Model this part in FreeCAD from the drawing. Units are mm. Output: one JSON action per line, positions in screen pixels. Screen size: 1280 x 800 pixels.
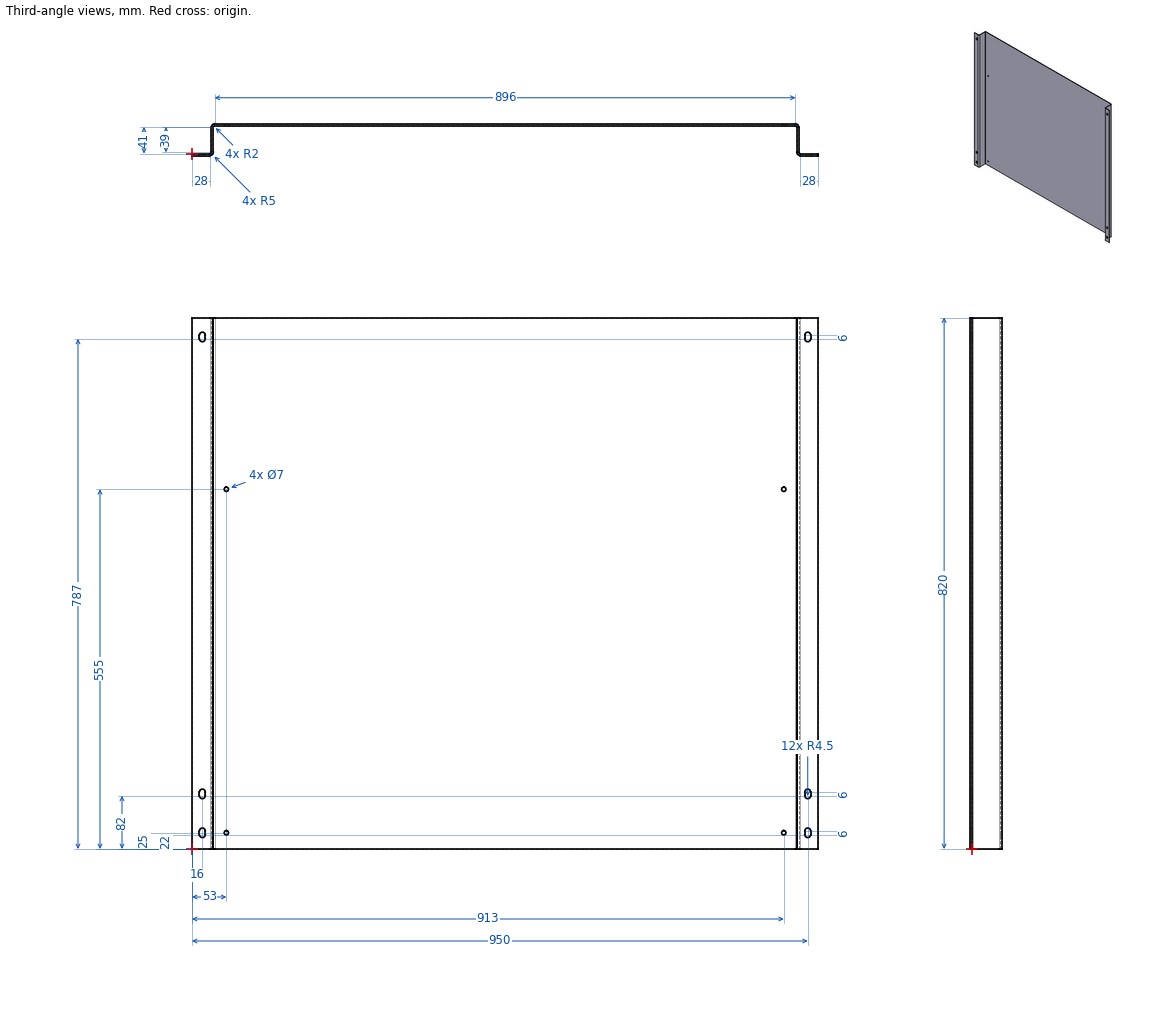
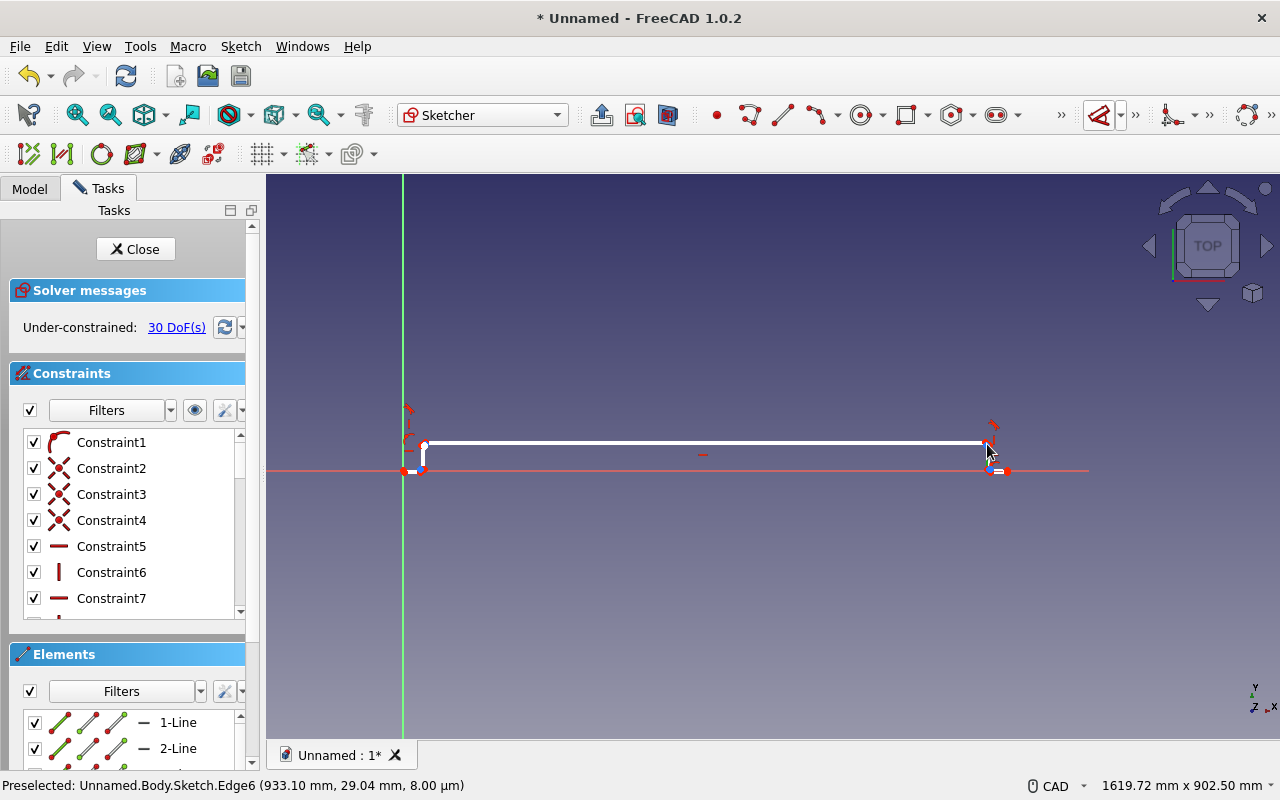
{"action": "scroll", "coordinate": [988, 471], "scroll_direction": "up", "scroll_amount": 12}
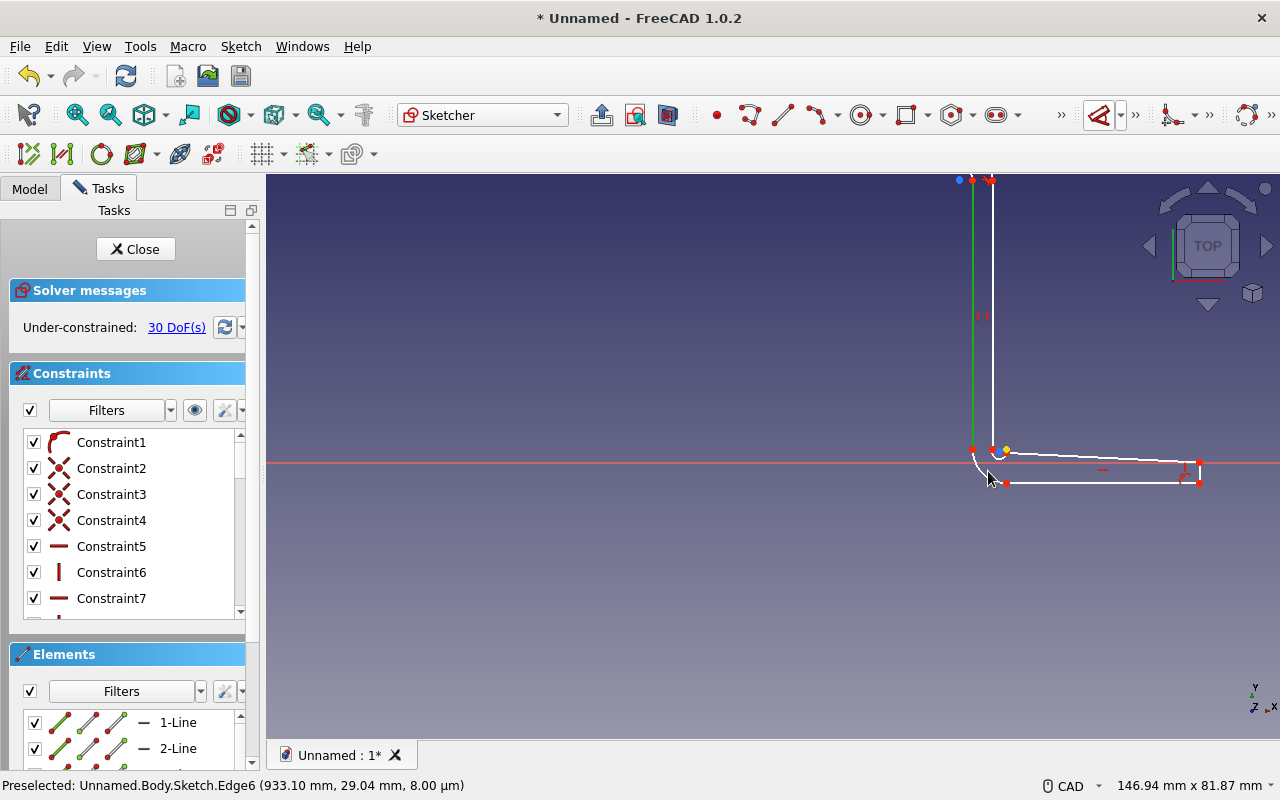
{"action": "left_click", "coordinate": [977, 465]}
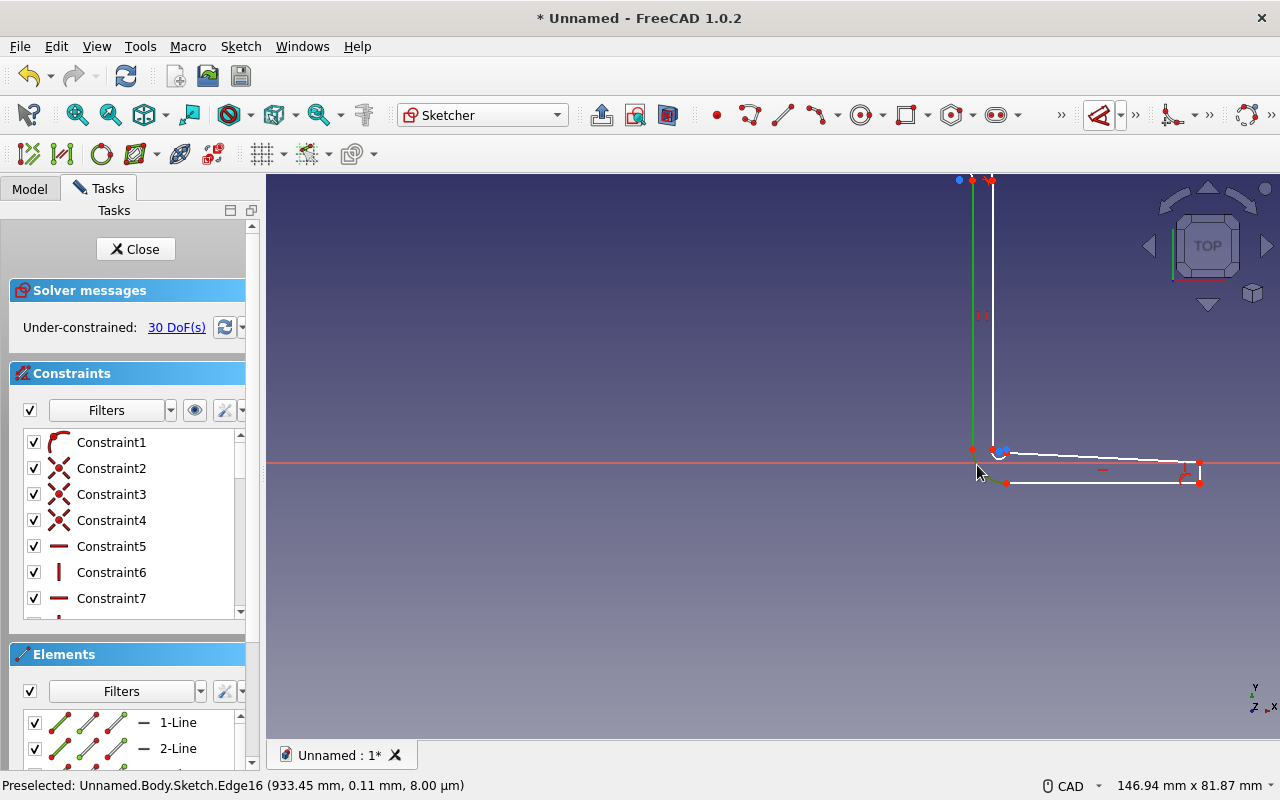
{"action": "key", "text": "t"}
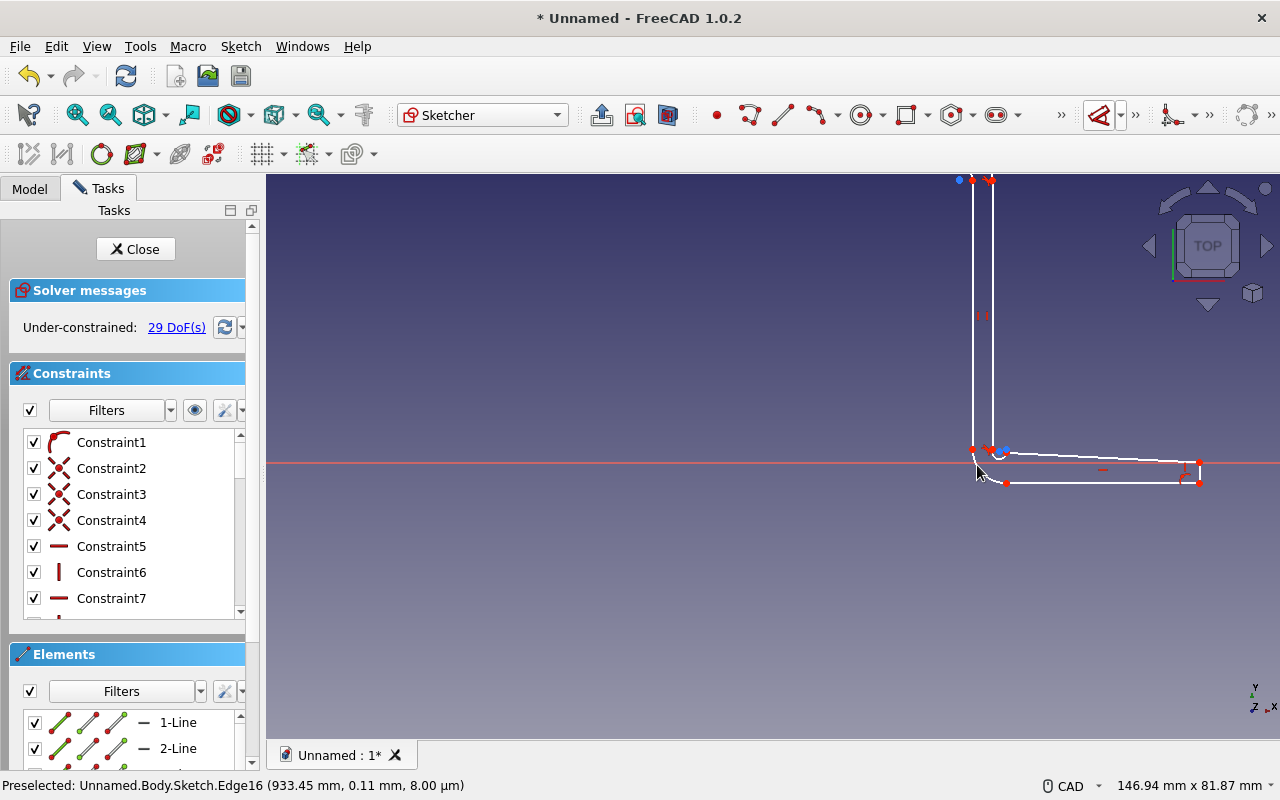
{"action": "left_click", "coordinate": [1064, 483]}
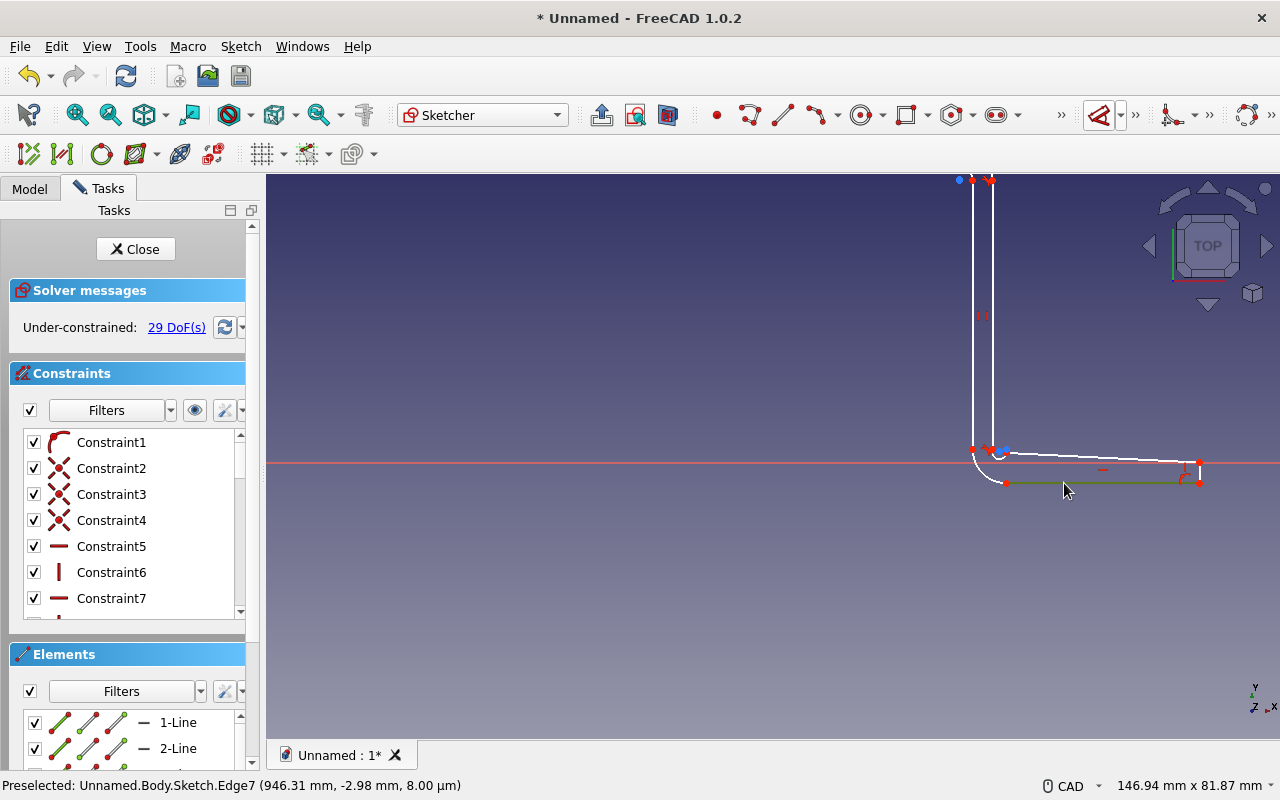
{"action": "left_click", "coordinate": [977, 465]}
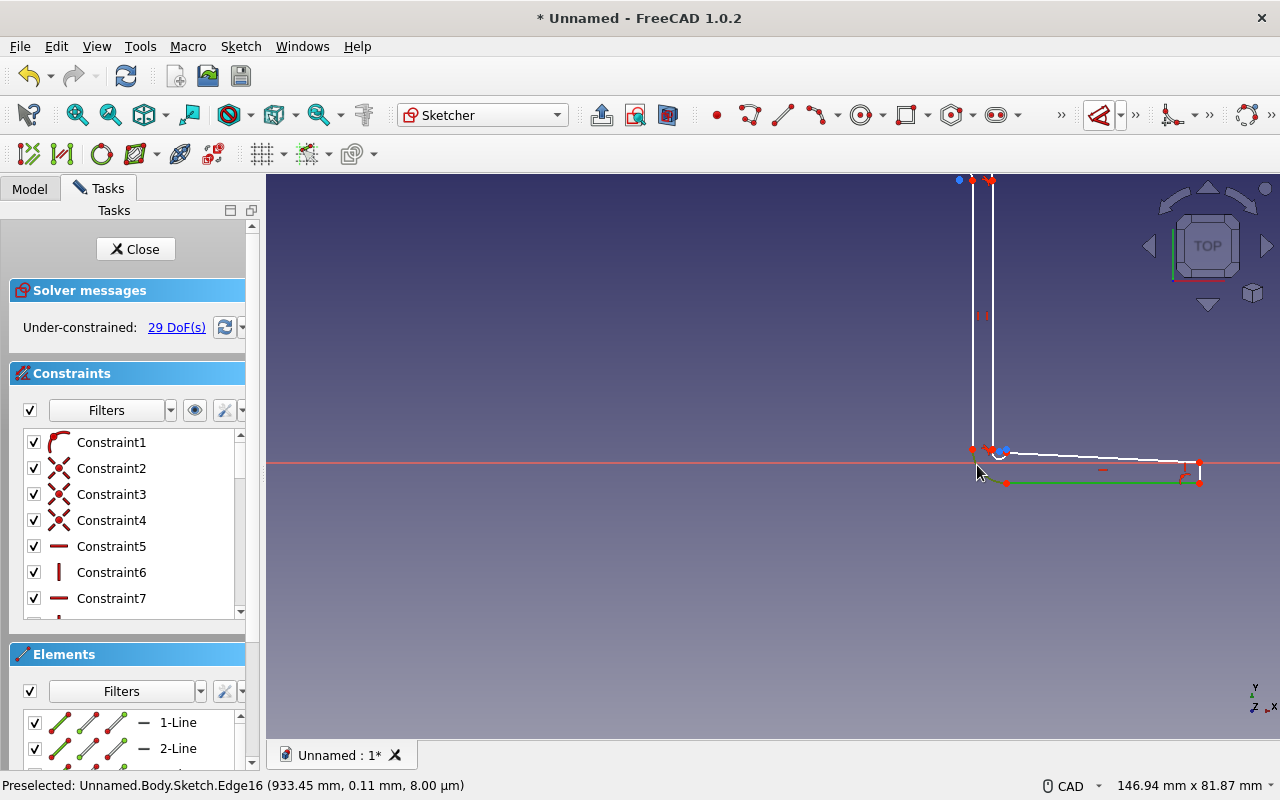
{"action": "key", "text": "t"}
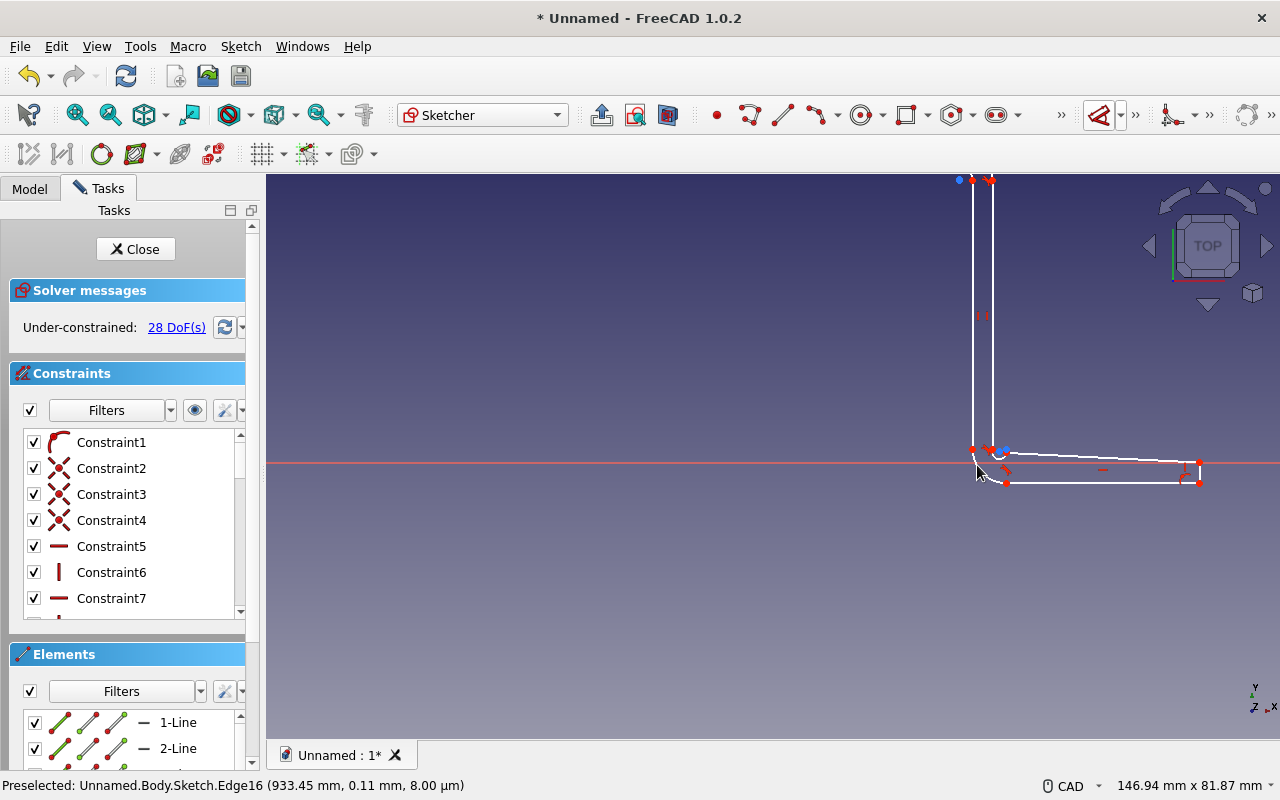
{"action": "scroll", "coordinate": [988, 471], "scroll_direction": "down", "scroll_amount": 12}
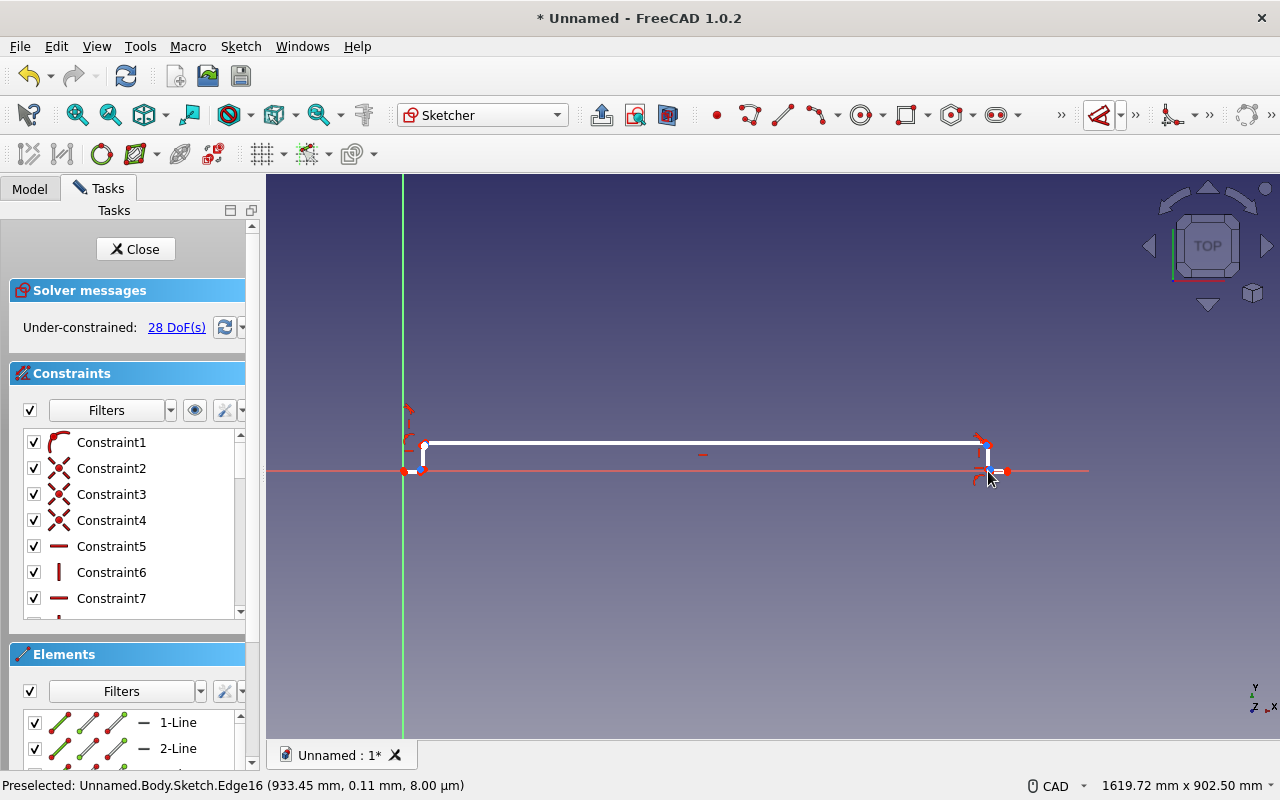
{"action": "scroll", "coordinate": [1003, 470], "scroll_direction": "up", "scroll_amount": 10}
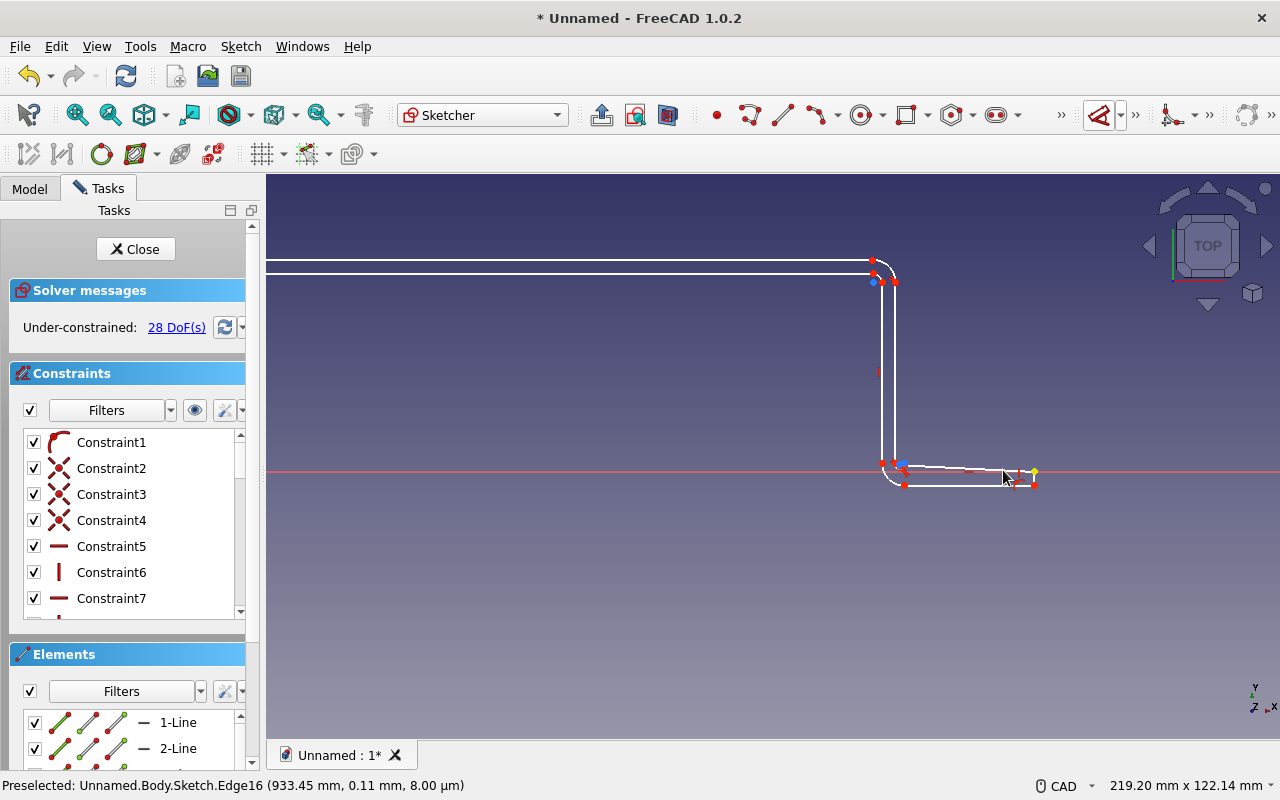
{"action": "left_click", "coordinate": [995, 470]}